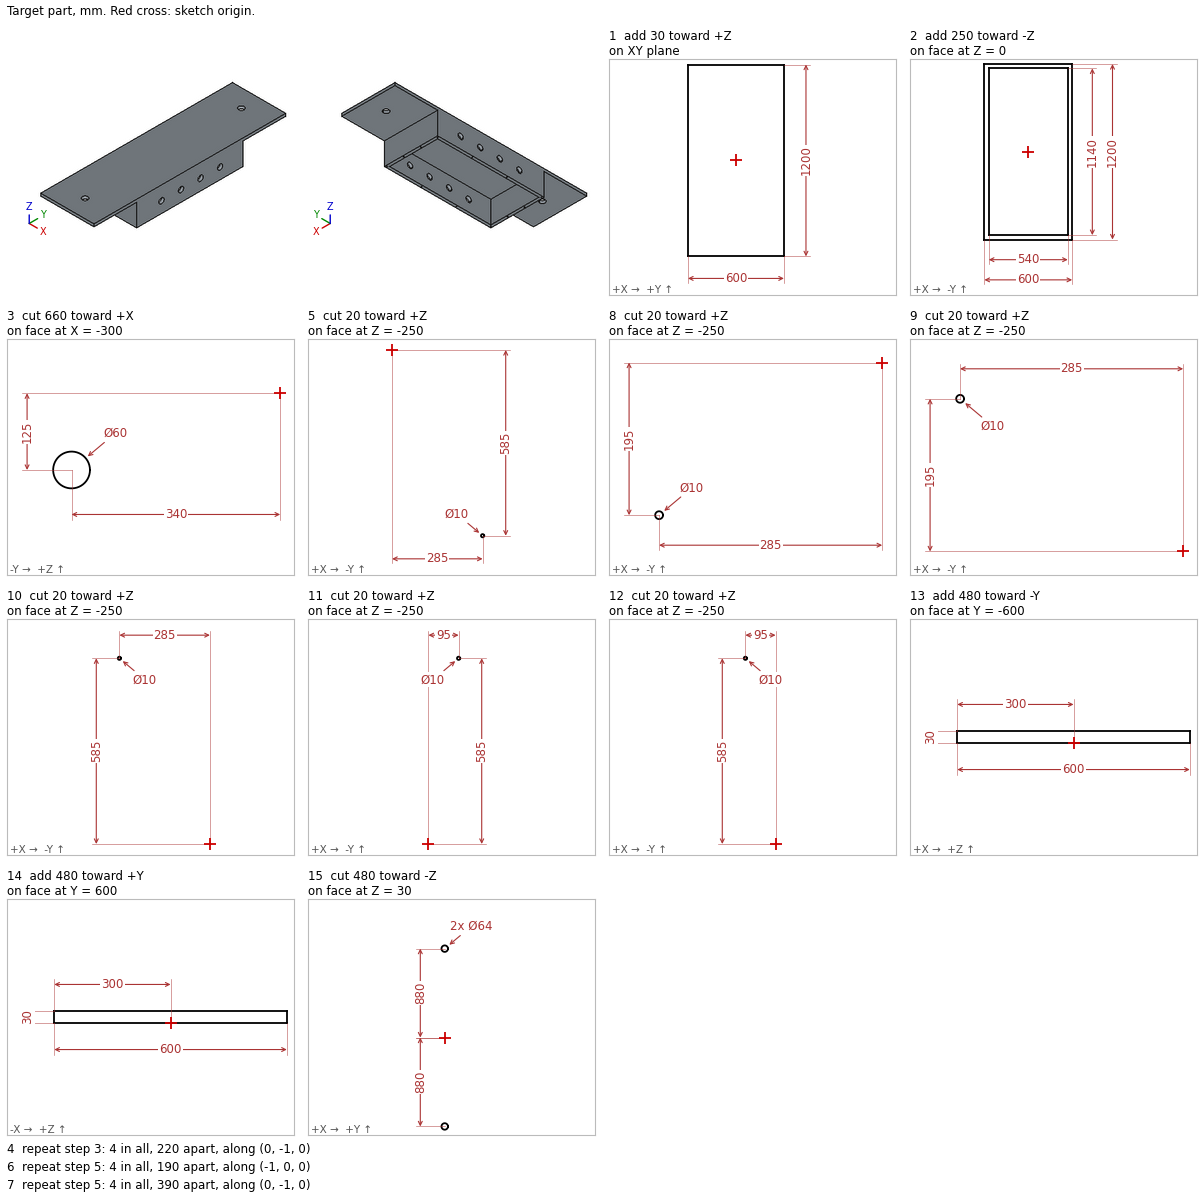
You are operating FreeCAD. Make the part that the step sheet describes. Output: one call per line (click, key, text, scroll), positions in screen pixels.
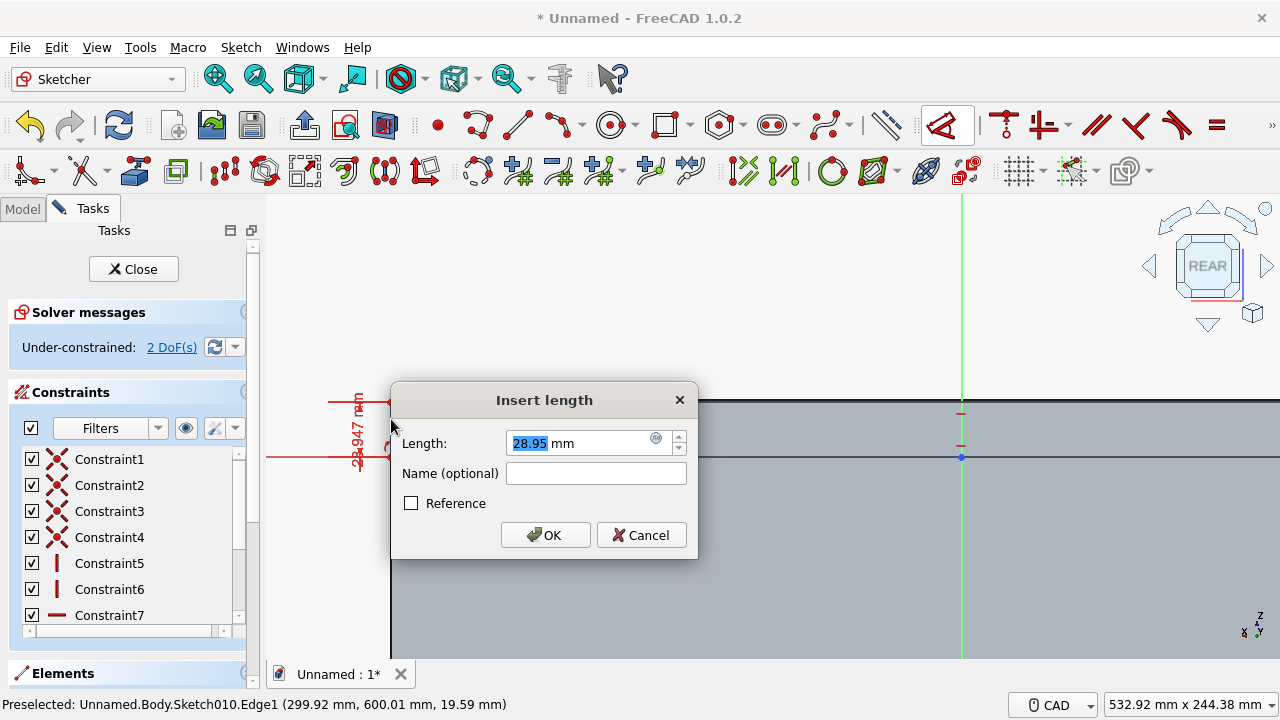
text(30)
key(Return)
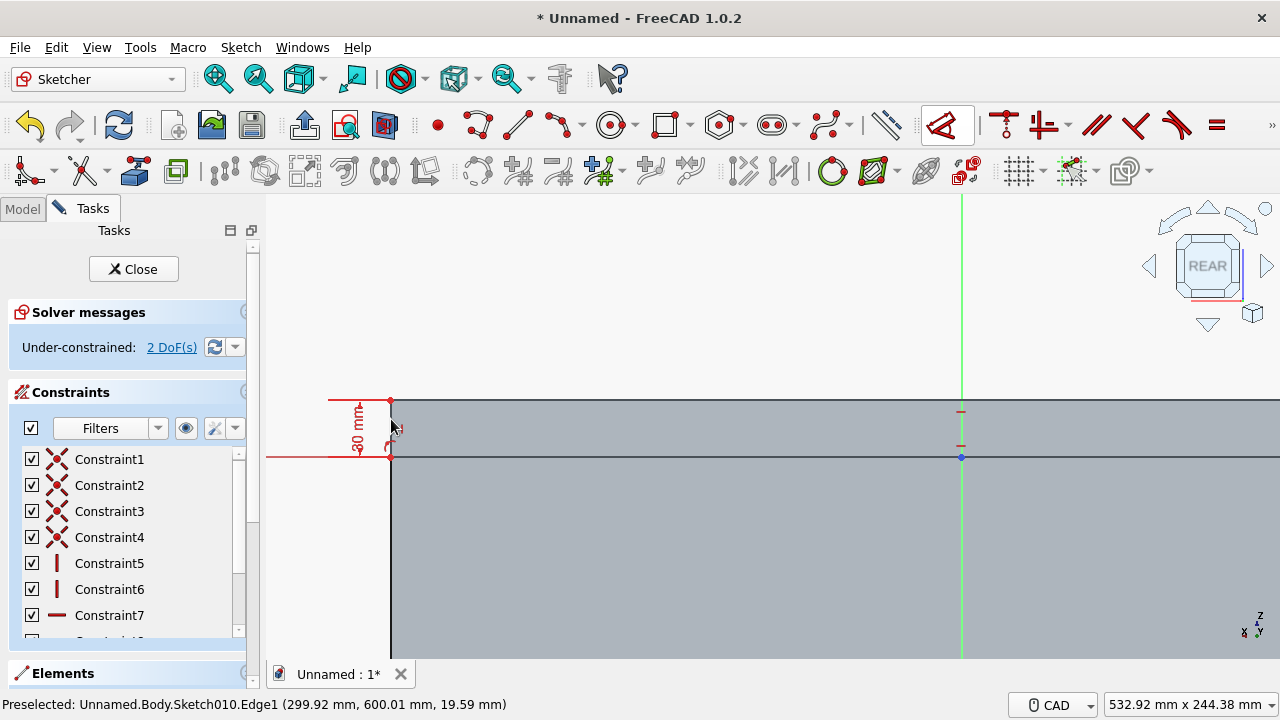
click(733, 457)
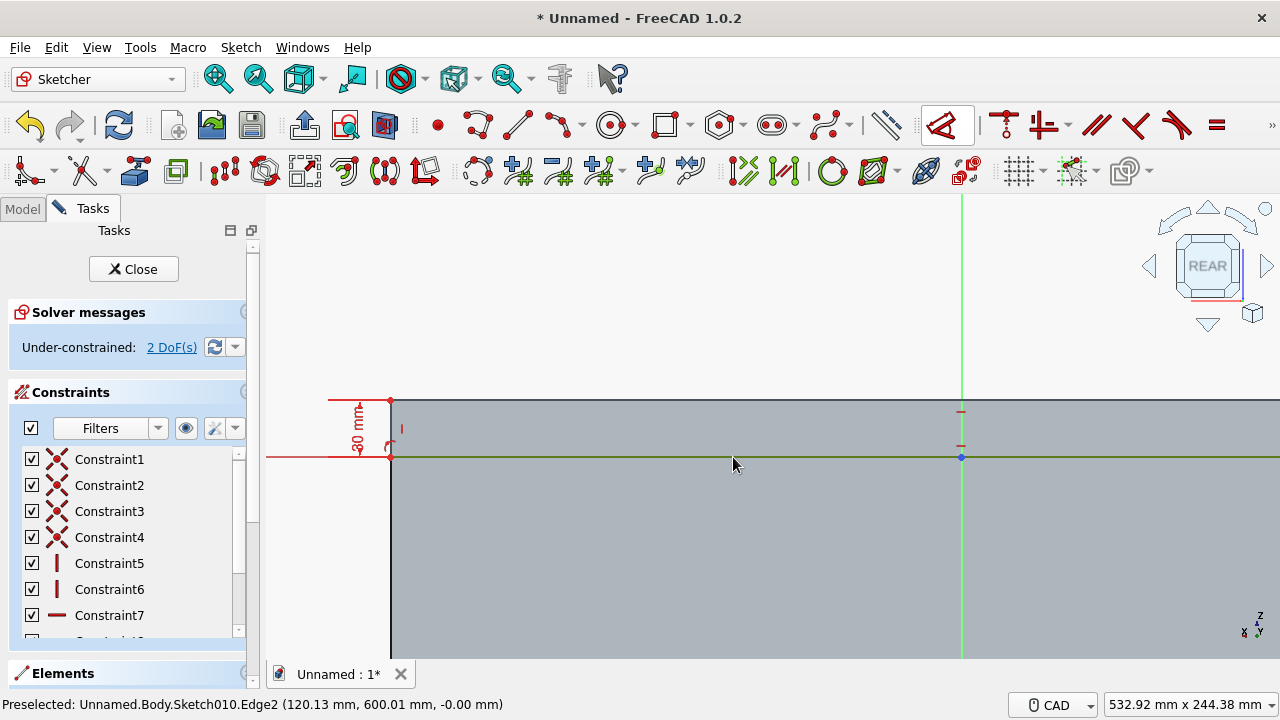
key(l)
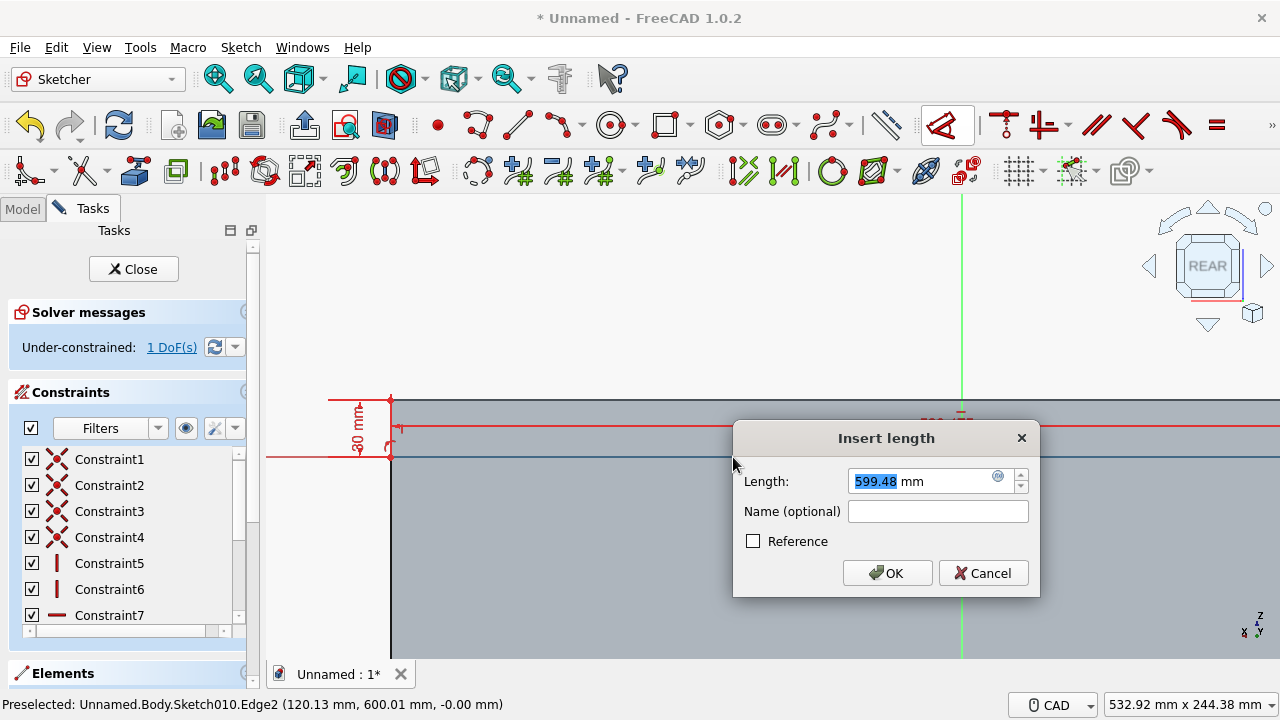
text(600)
key(Return)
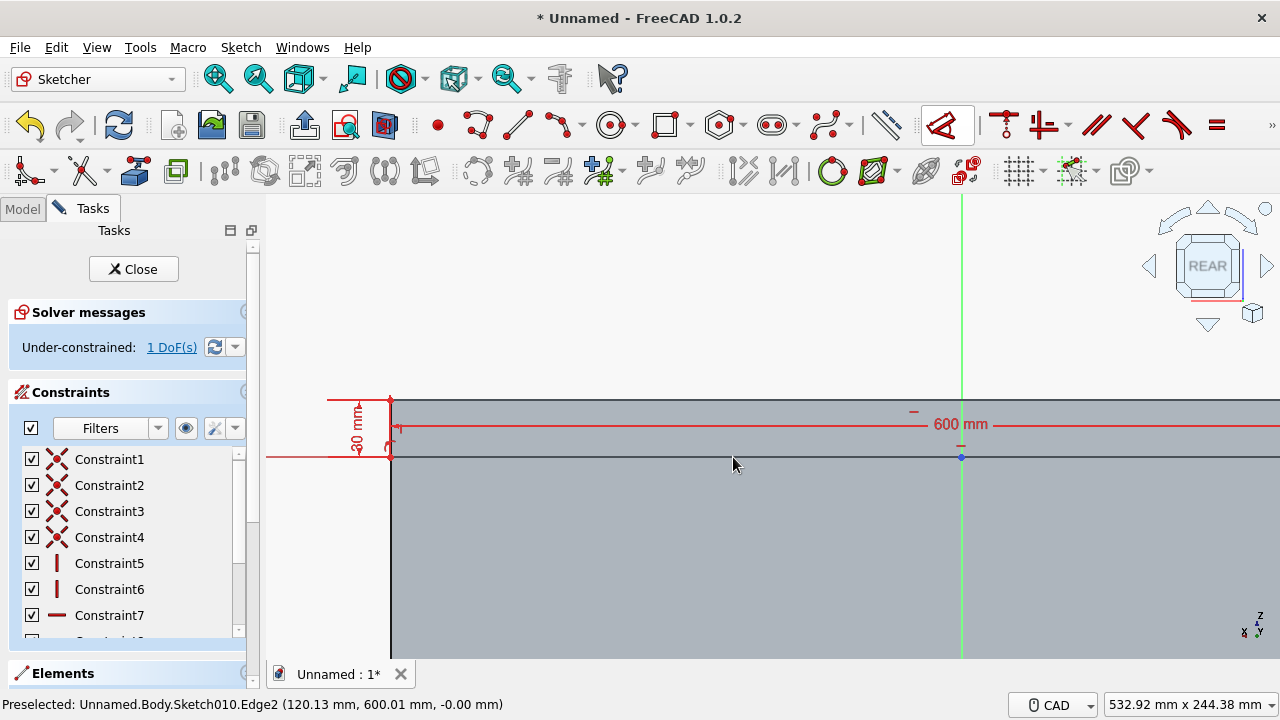
click(390, 400)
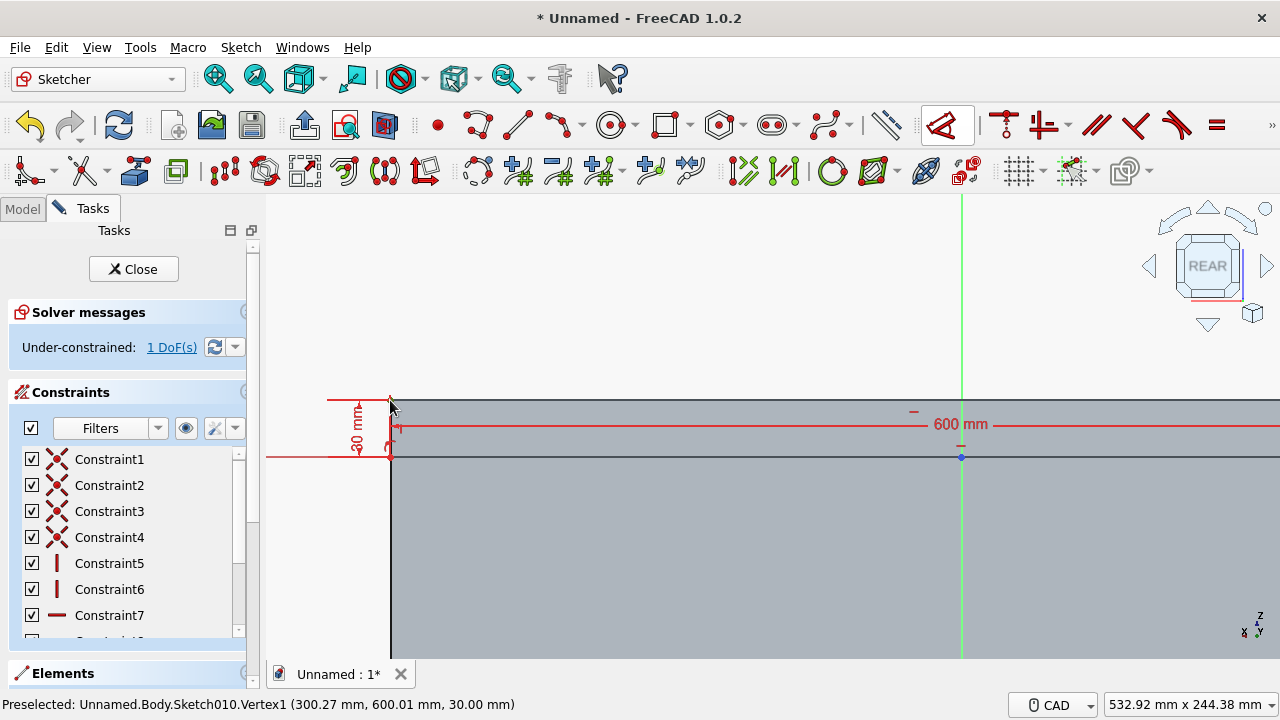
click(968, 126)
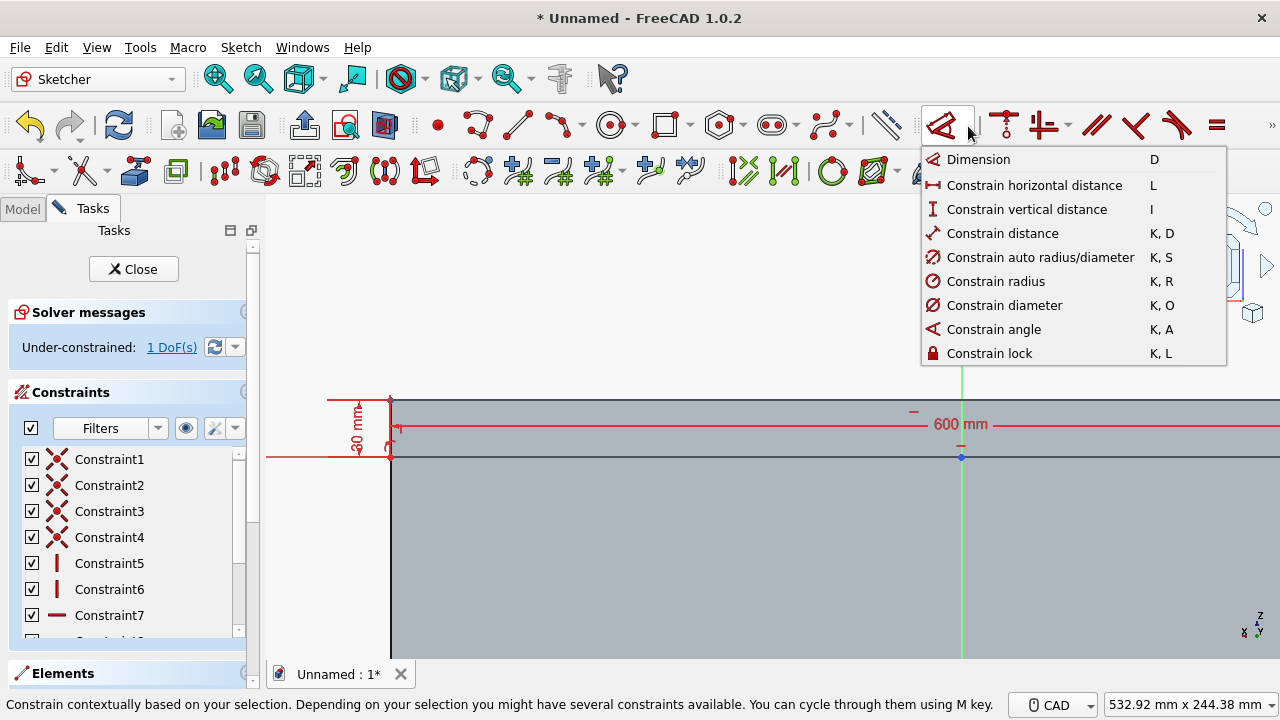
click(1074, 185)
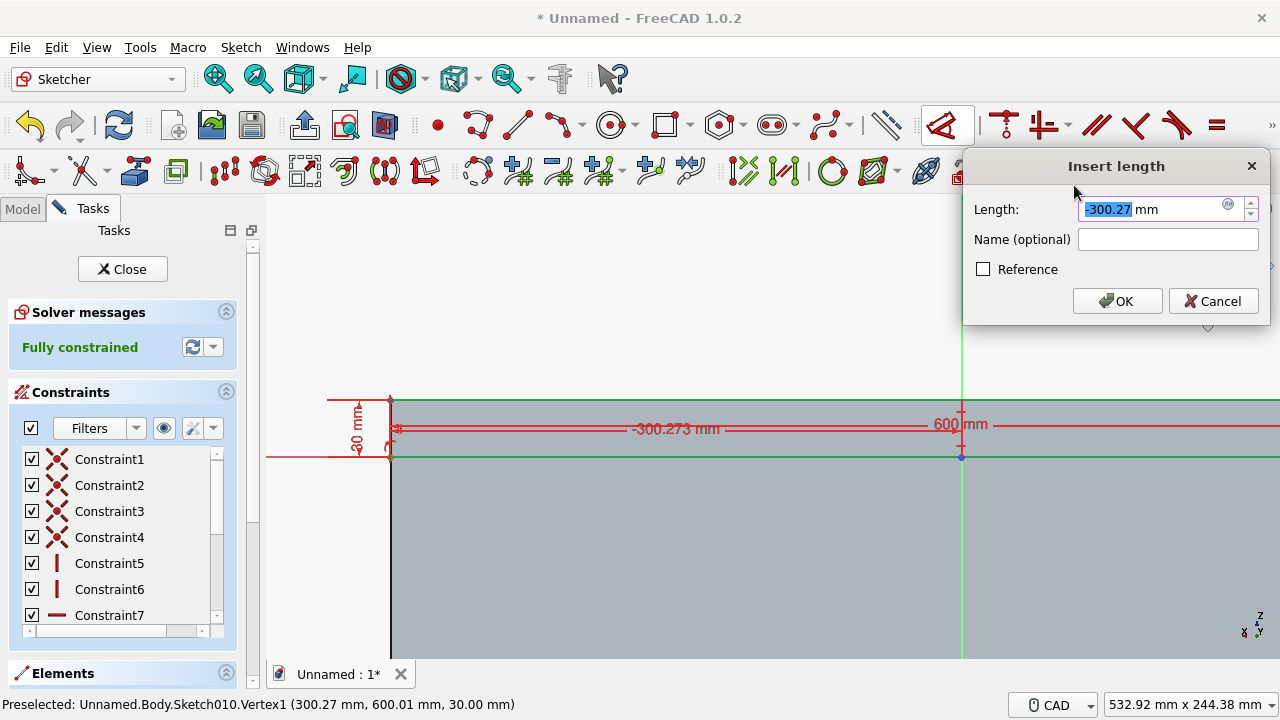
text(-300)
key(Return)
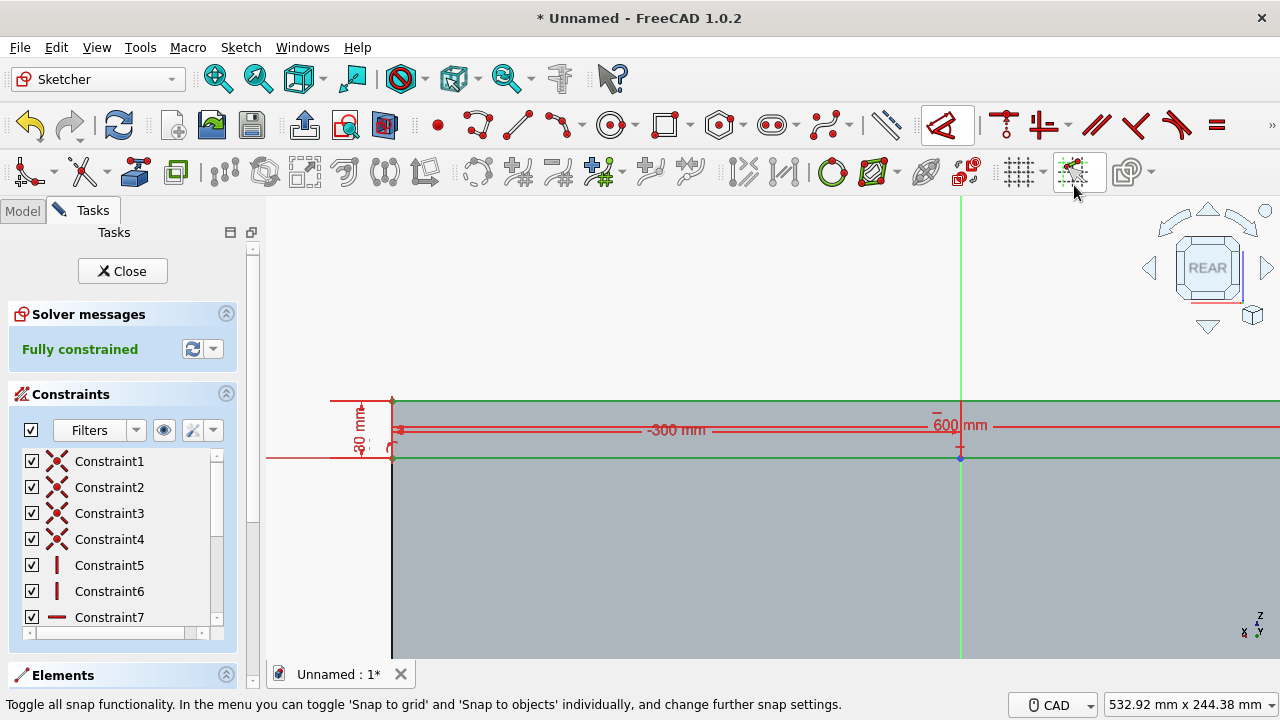
click(123, 271)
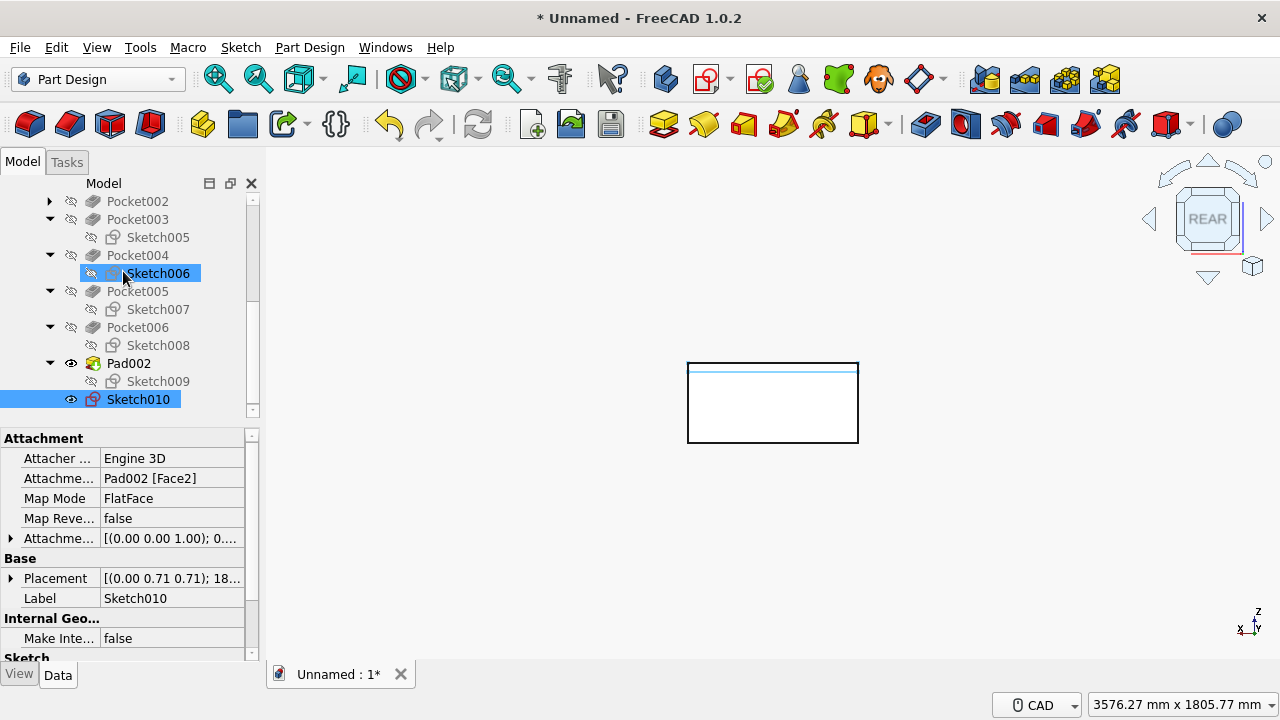
click(664, 124)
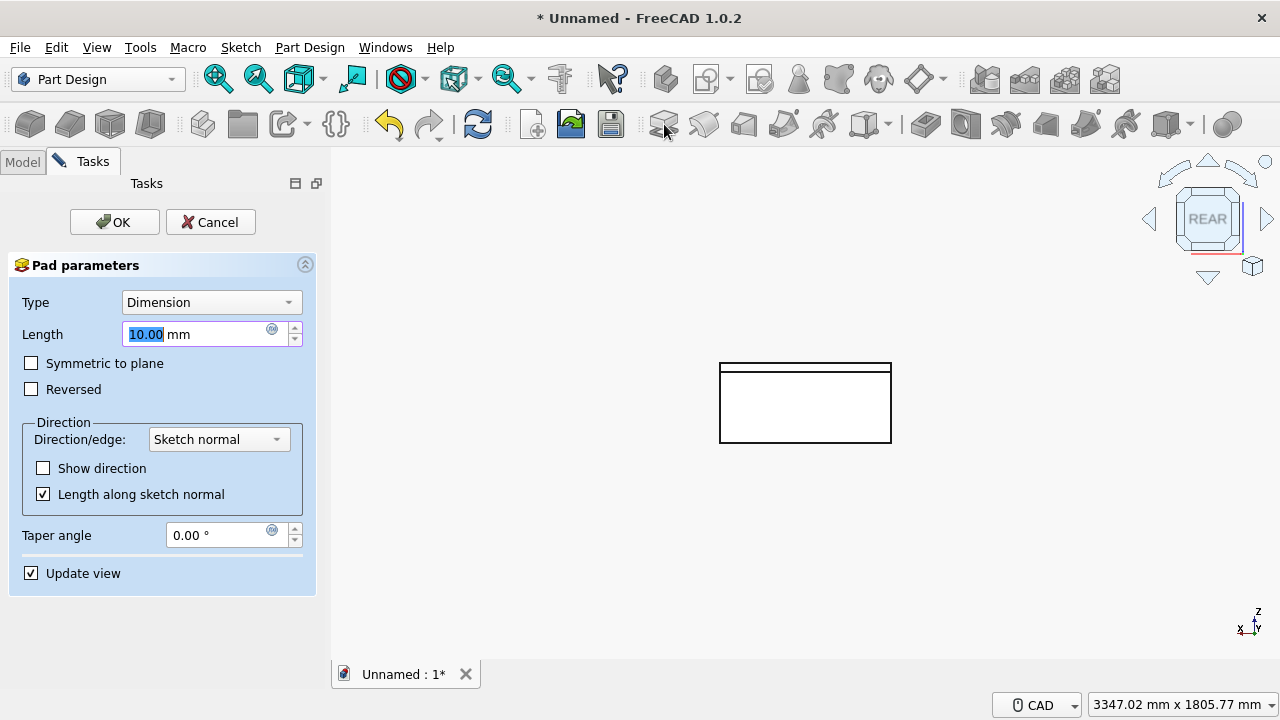
text(480)
key(Tab)